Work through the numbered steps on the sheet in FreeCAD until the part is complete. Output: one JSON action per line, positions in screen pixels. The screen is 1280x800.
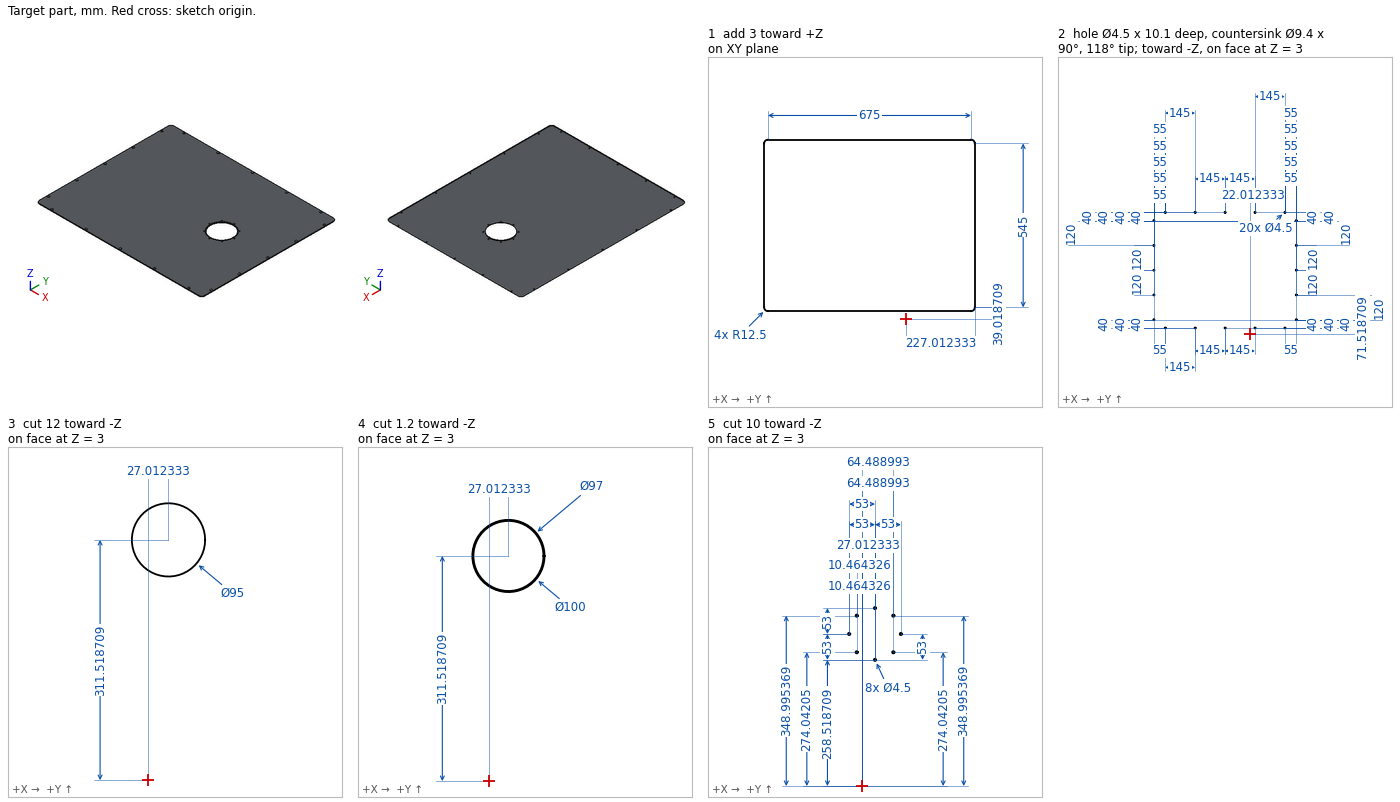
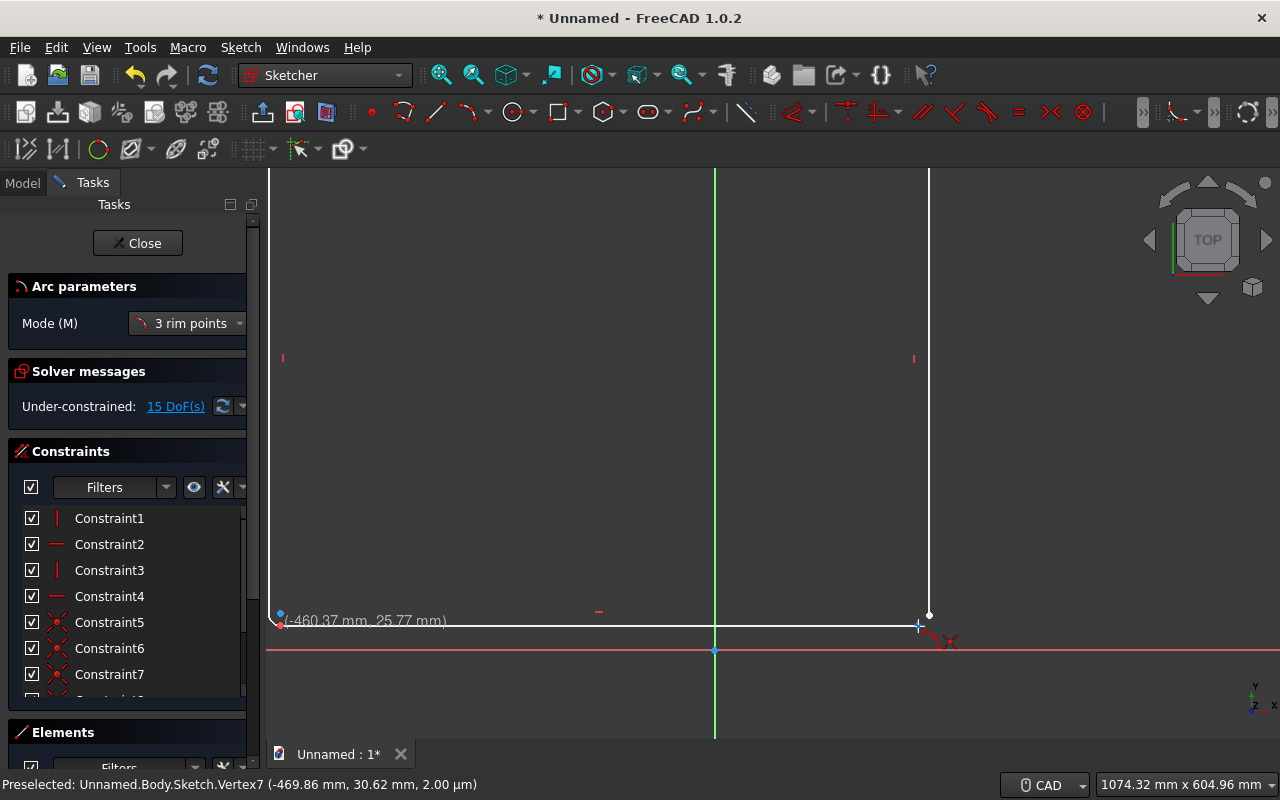
{"action": "left_click", "coordinate": [918, 626]}
{"action": "left_click", "coordinate": [929, 616]}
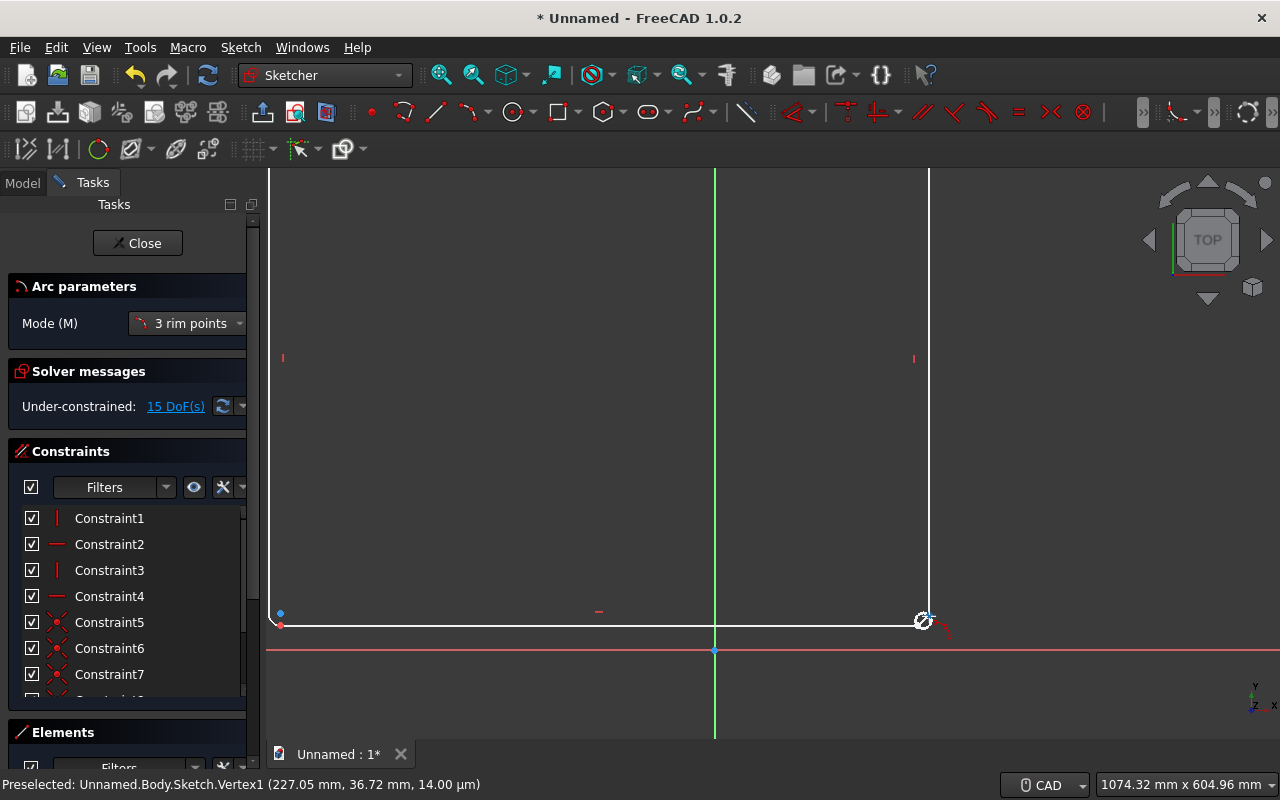
{"action": "scroll", "coordinate": [926, 622], "scroll_direction": "up", "scroll_amount": 8}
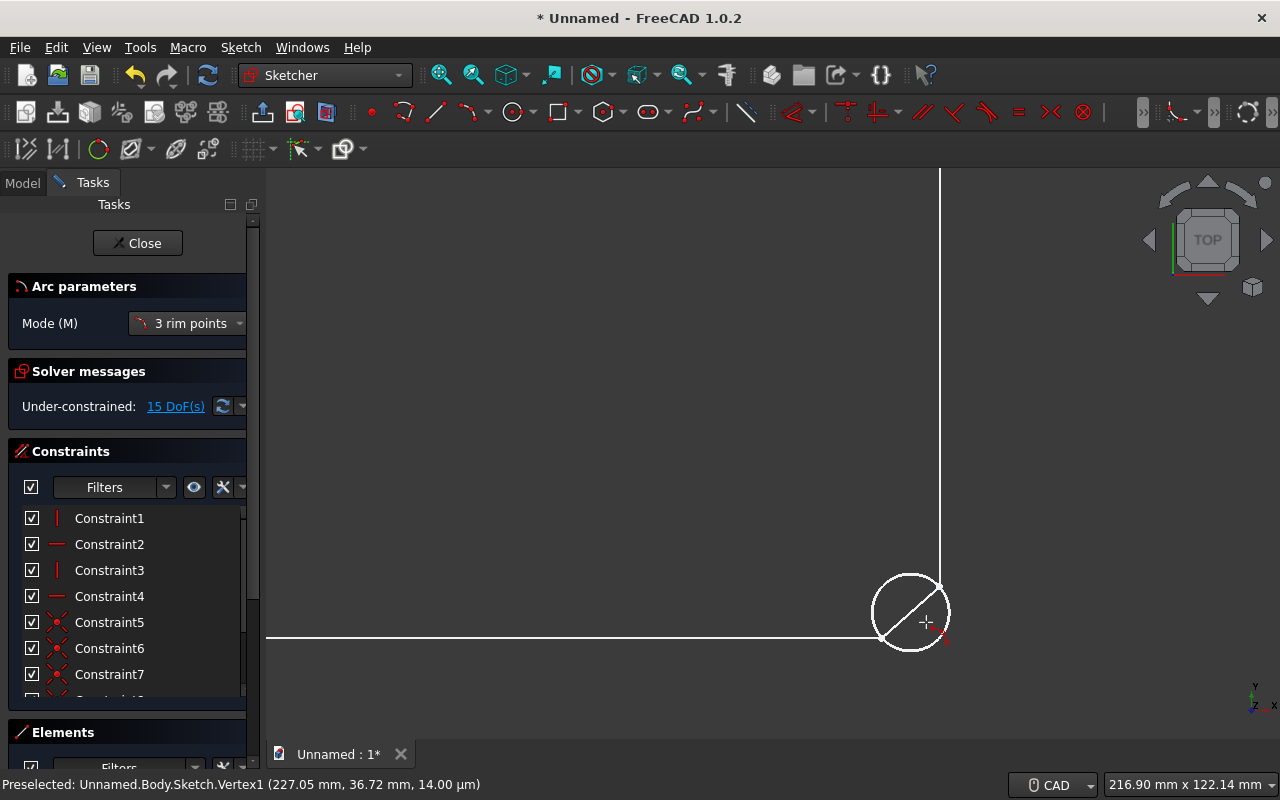
{"action": "left_click", "coordinate": [922, 617]}
{"action": "key", "text": "Escape"}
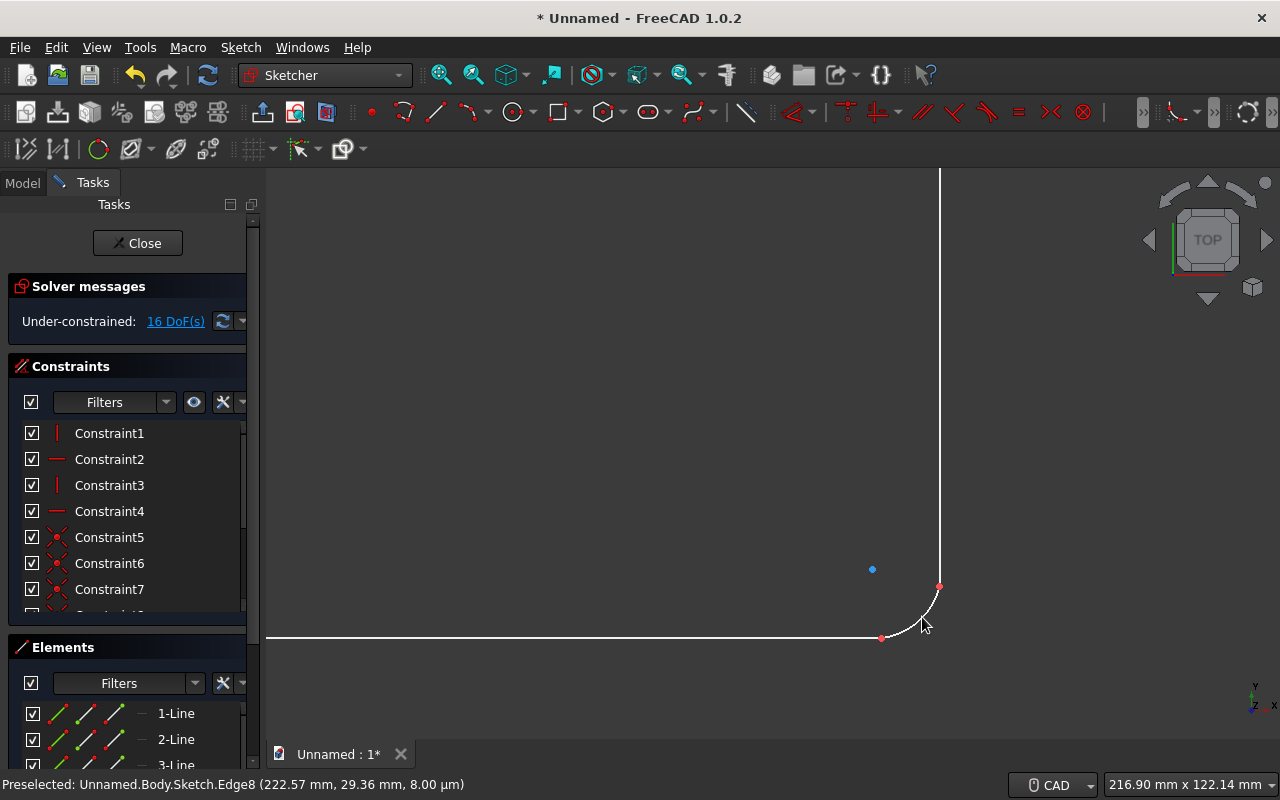
{"action": "scroll", "coordinate": [924, 624], "scroll_direction": "down", "scroll_amount": 10}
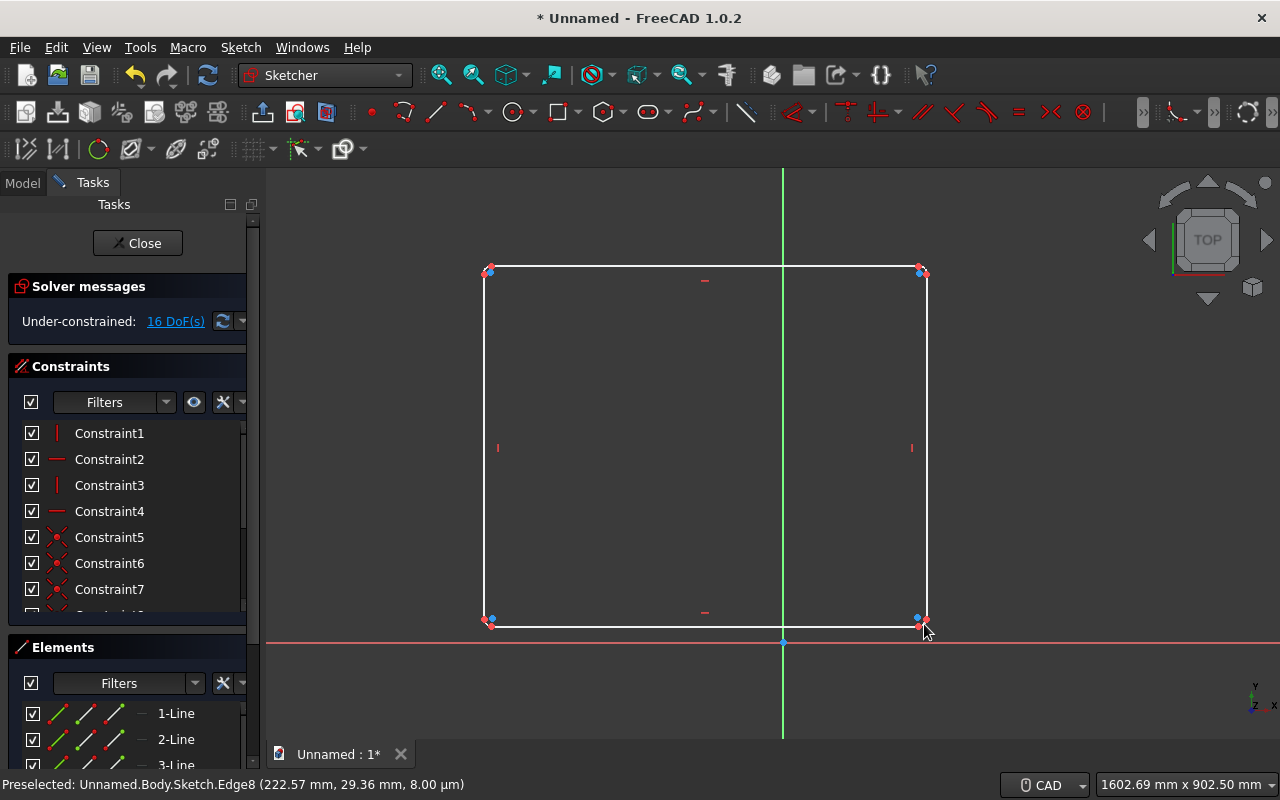
{"action": "left_click", "coordinate": [927, 516]}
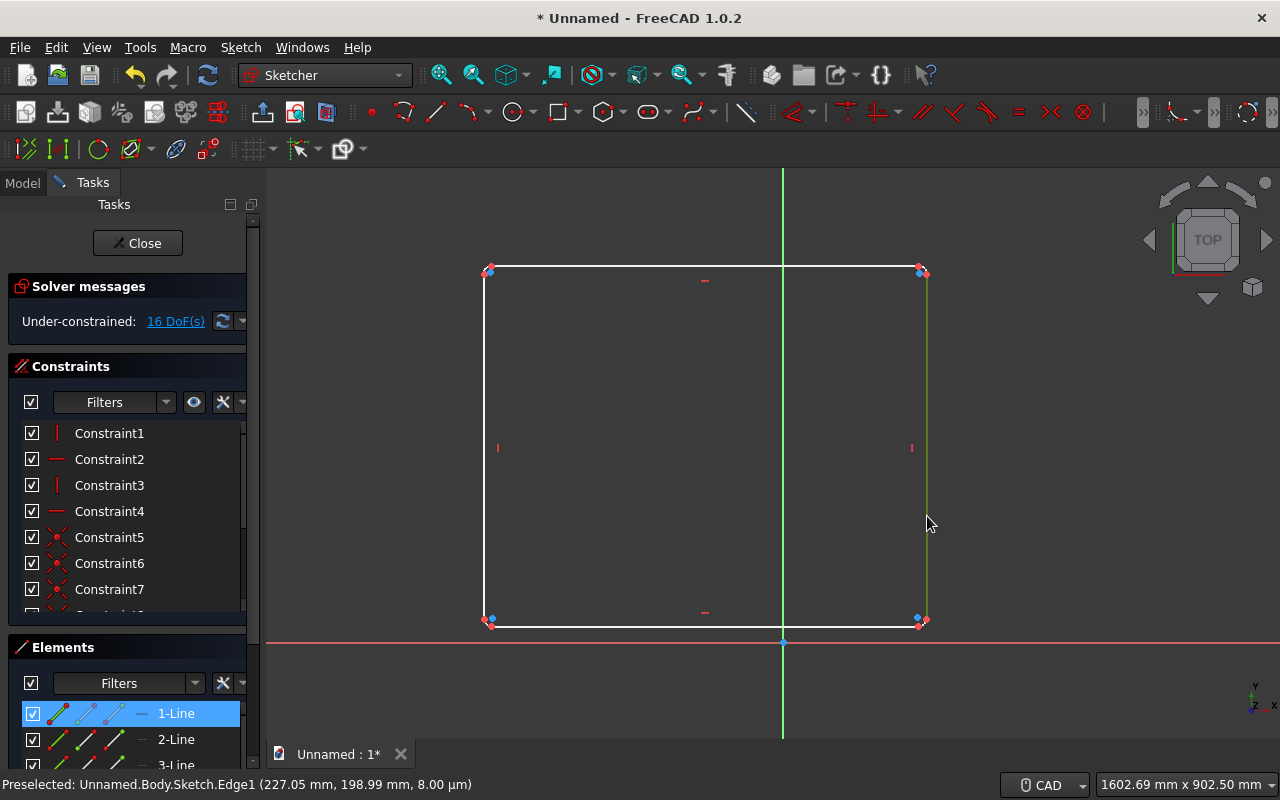
{"action": "scroll", "coordinate": [925, 269], "scroll_direction": "up", "scroll_amount": 4}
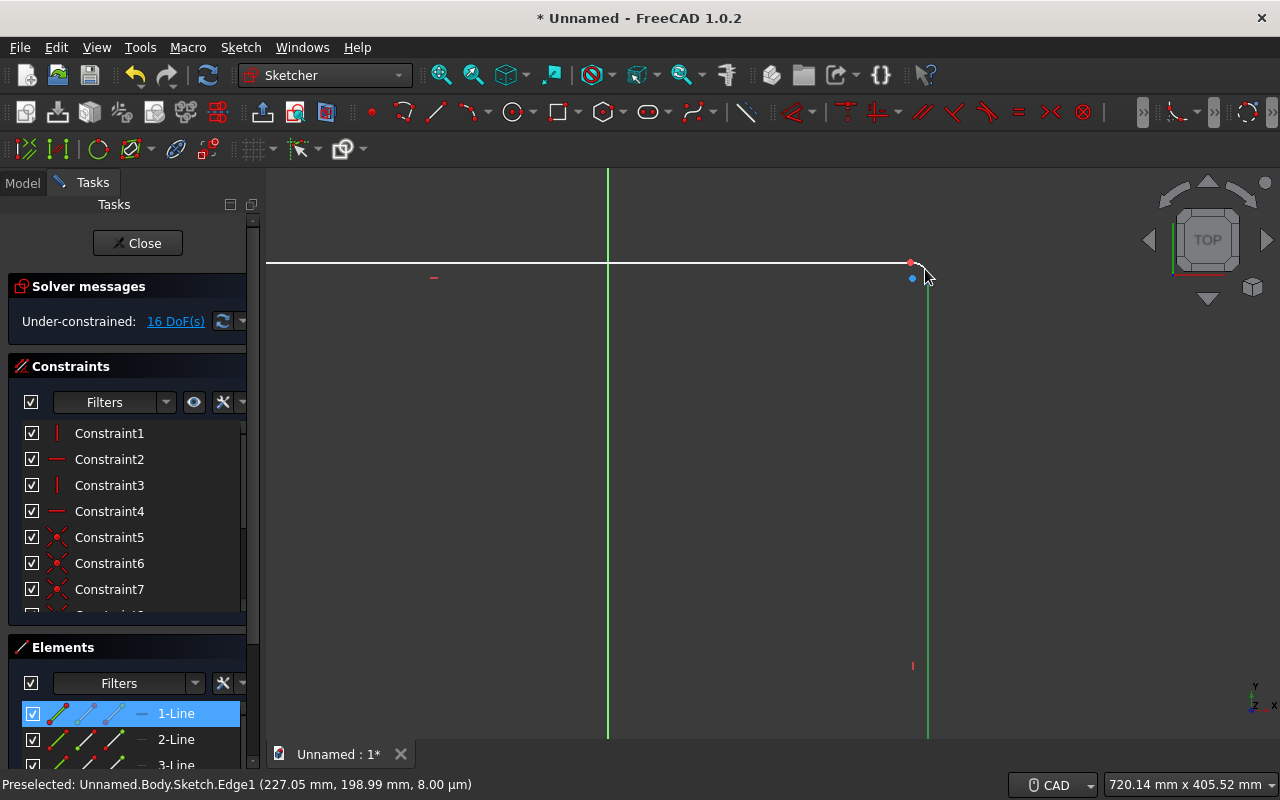
{"action": "left_click", "coordinate": [924, 268]}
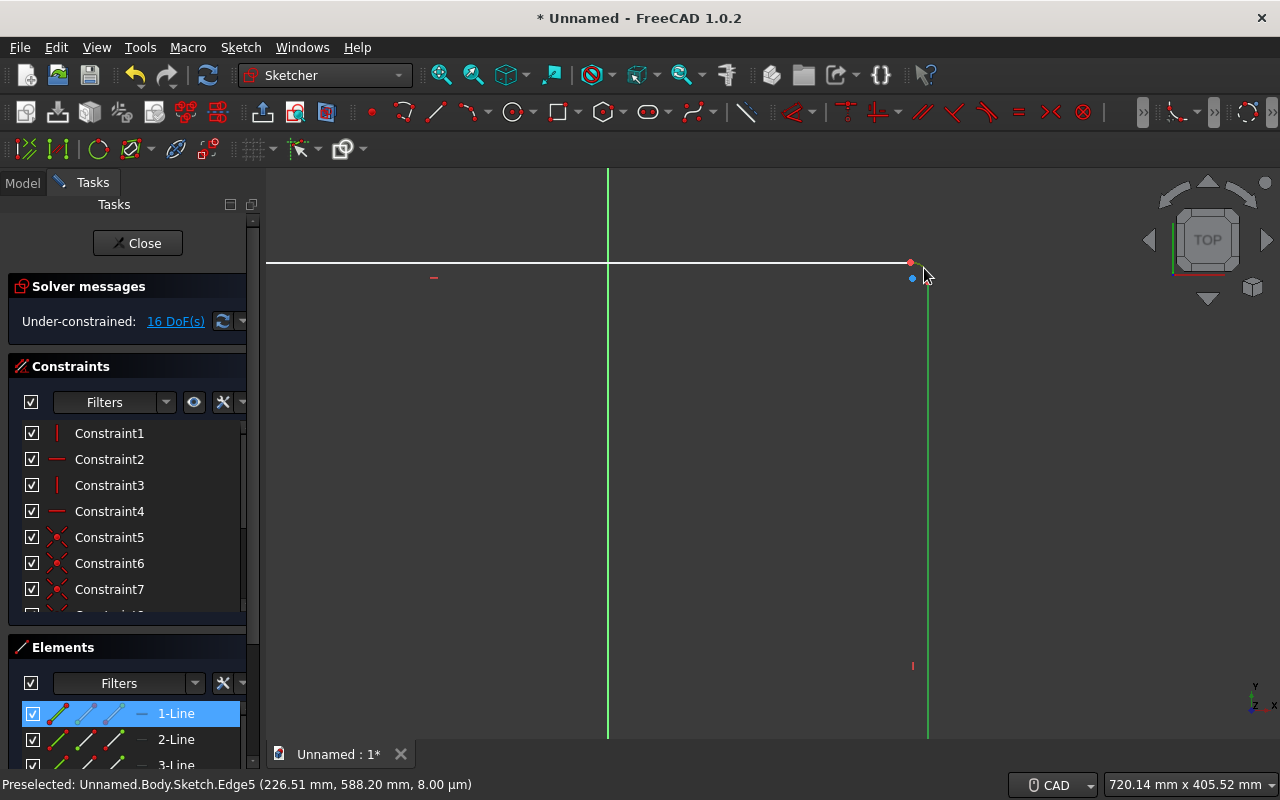
{"action": "left_click", "coordinate": [988, 112]}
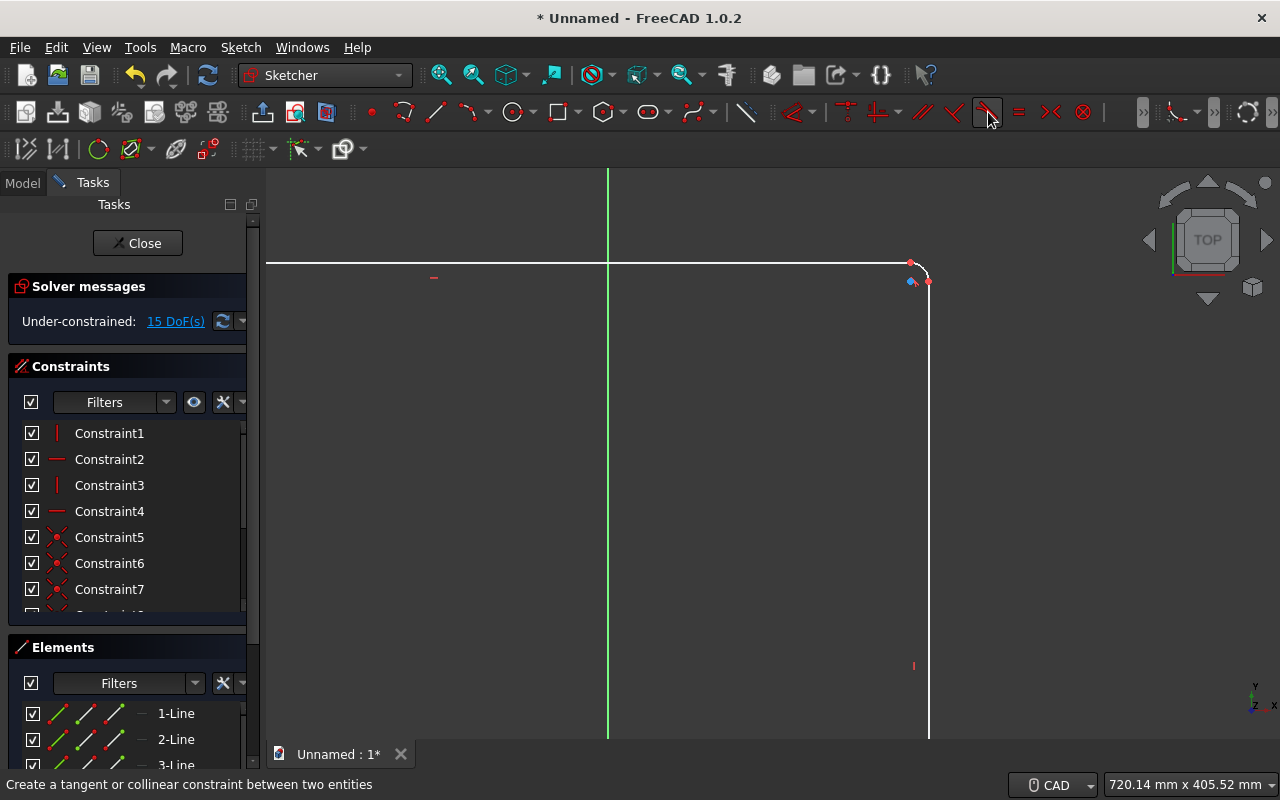
{"action": "left_click", "coordinate": [929, 512]}